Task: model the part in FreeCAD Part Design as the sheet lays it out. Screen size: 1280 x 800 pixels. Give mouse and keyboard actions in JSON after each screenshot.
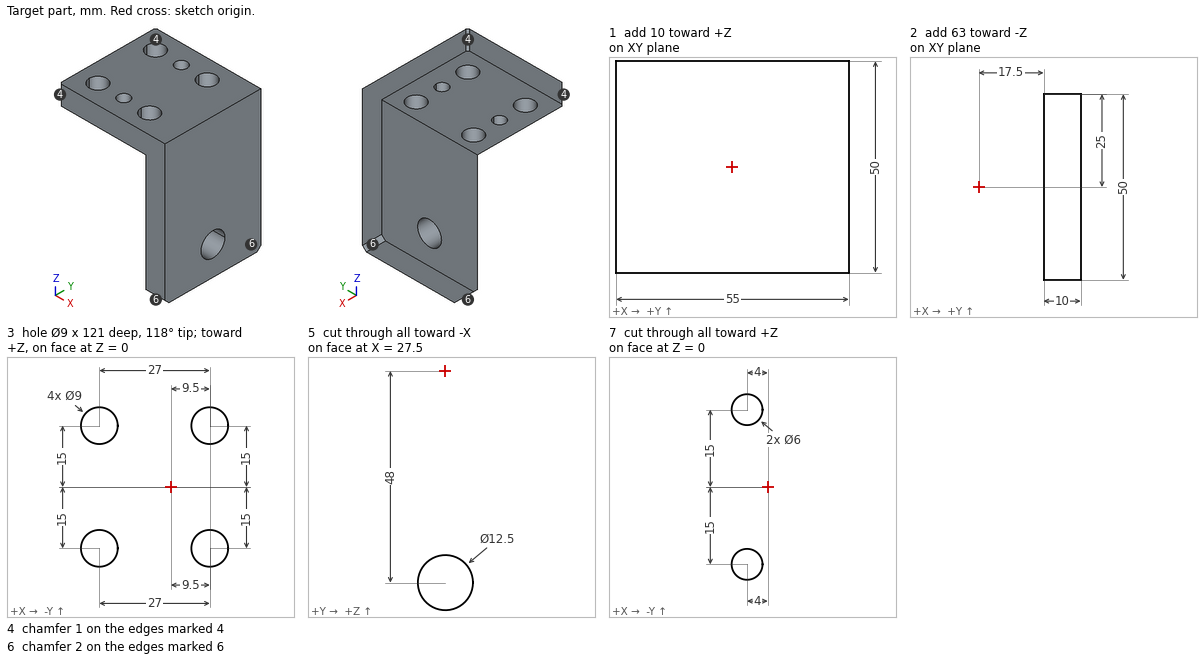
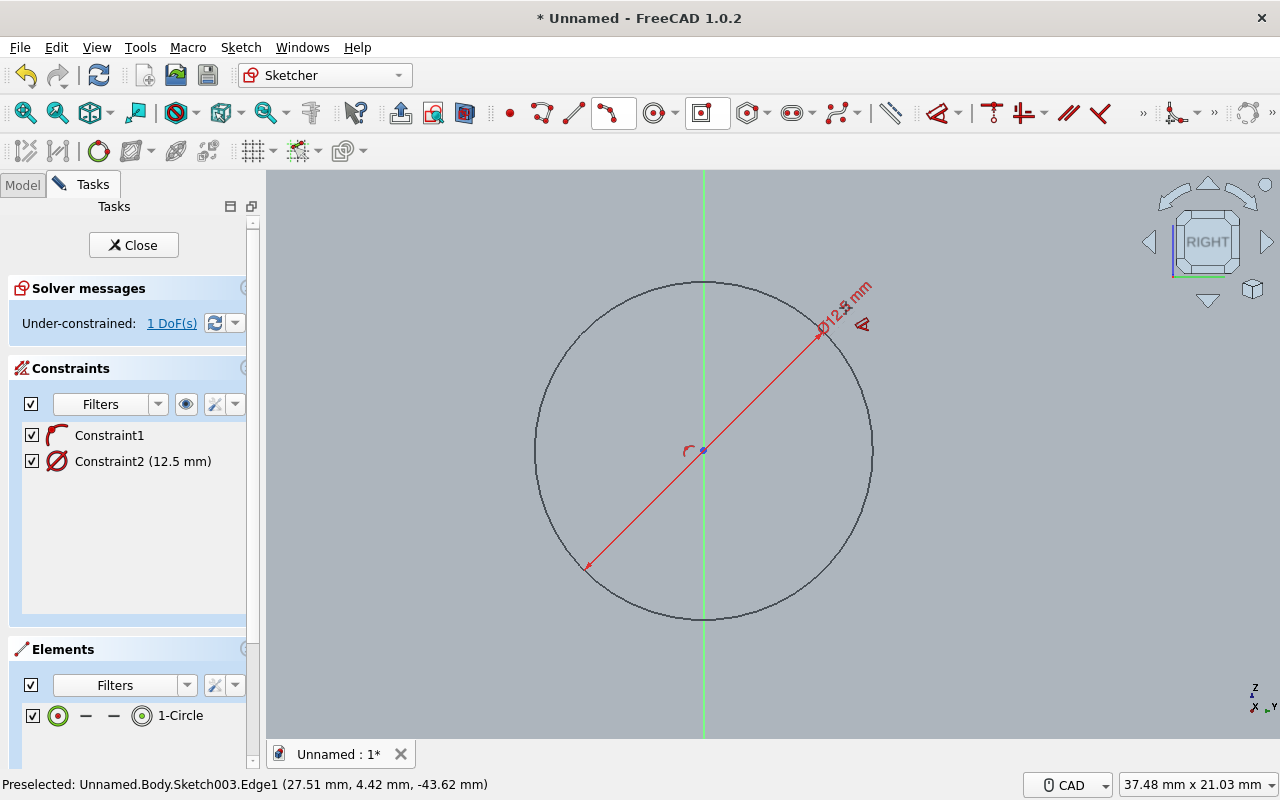
{"action": "left_click", "coordinate": [704, 451]}
{"action": "left_click", "coordinate": [738, 325]}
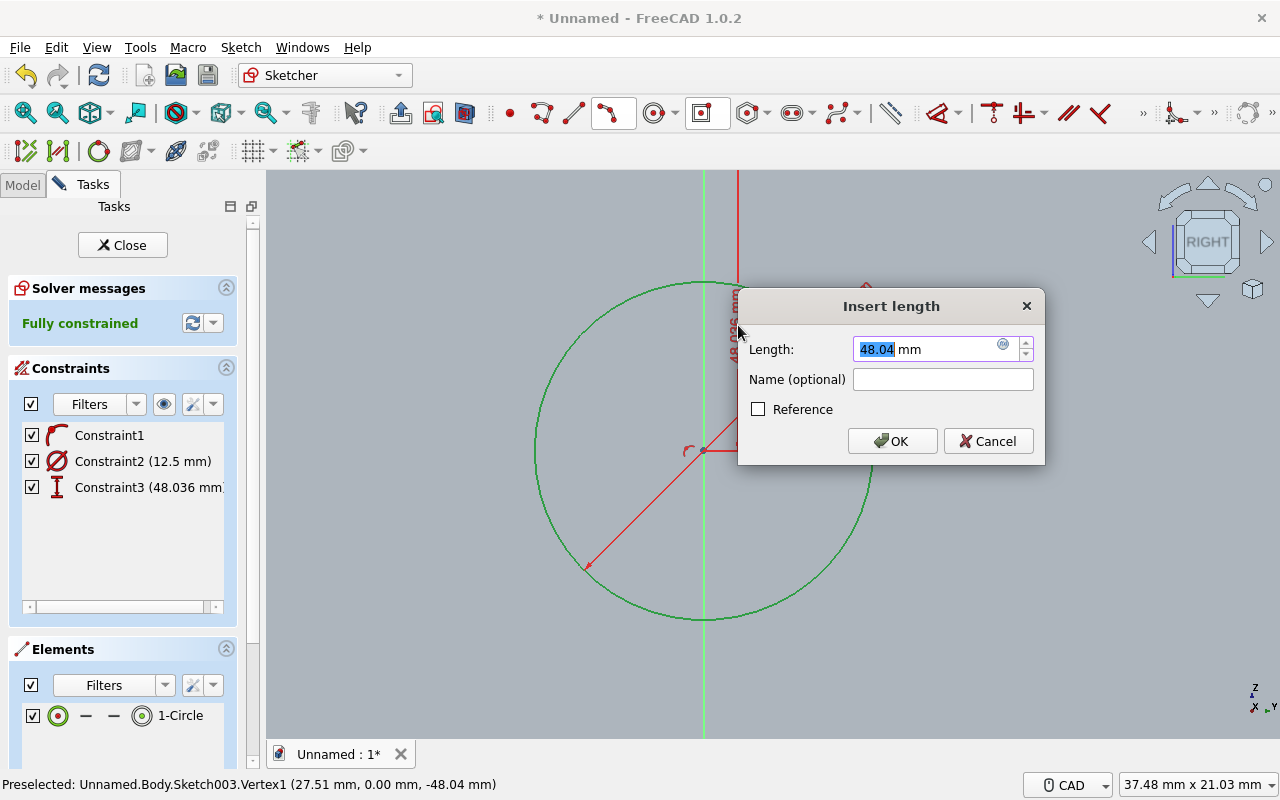
{"action": "type", "text": "48"}
{"action": "key", "text": "Return"}
{"action": "key", "text": "Escape"}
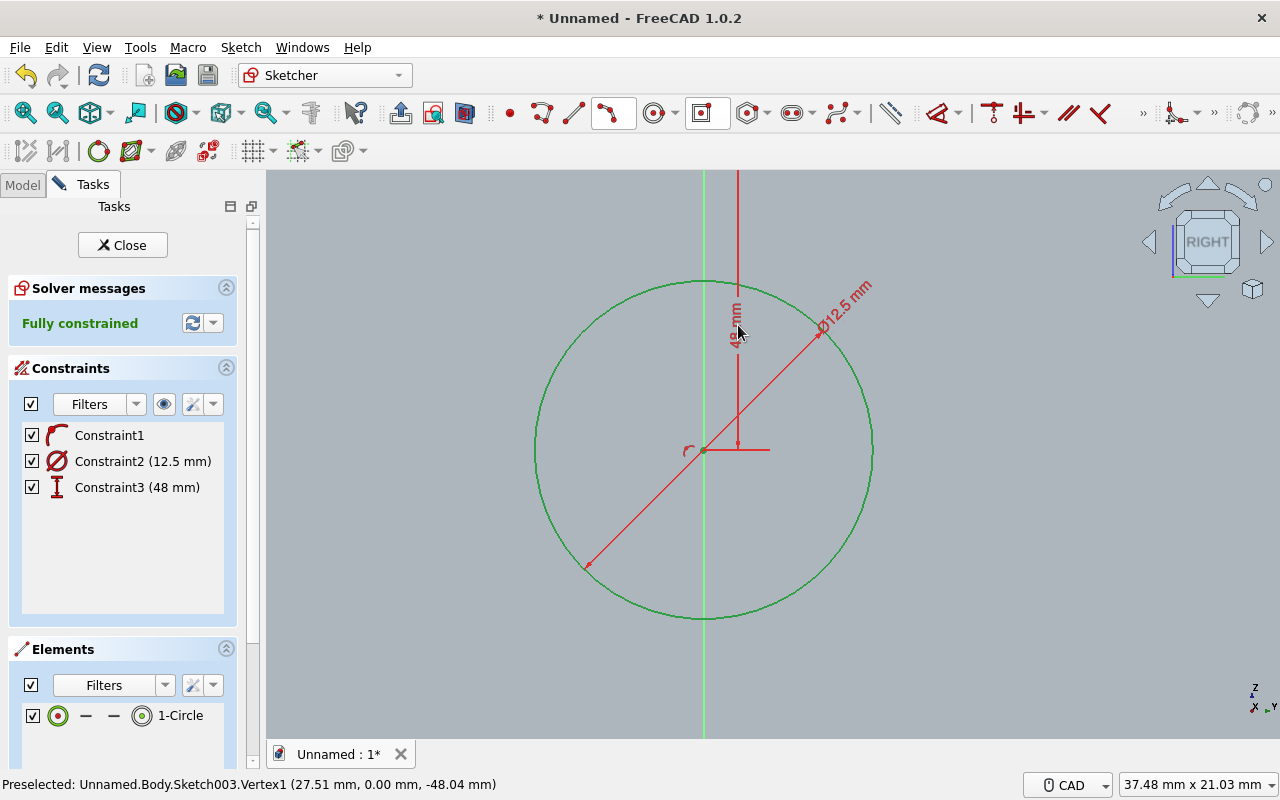
{"action": "left_click", "coordinate": [123, 245]}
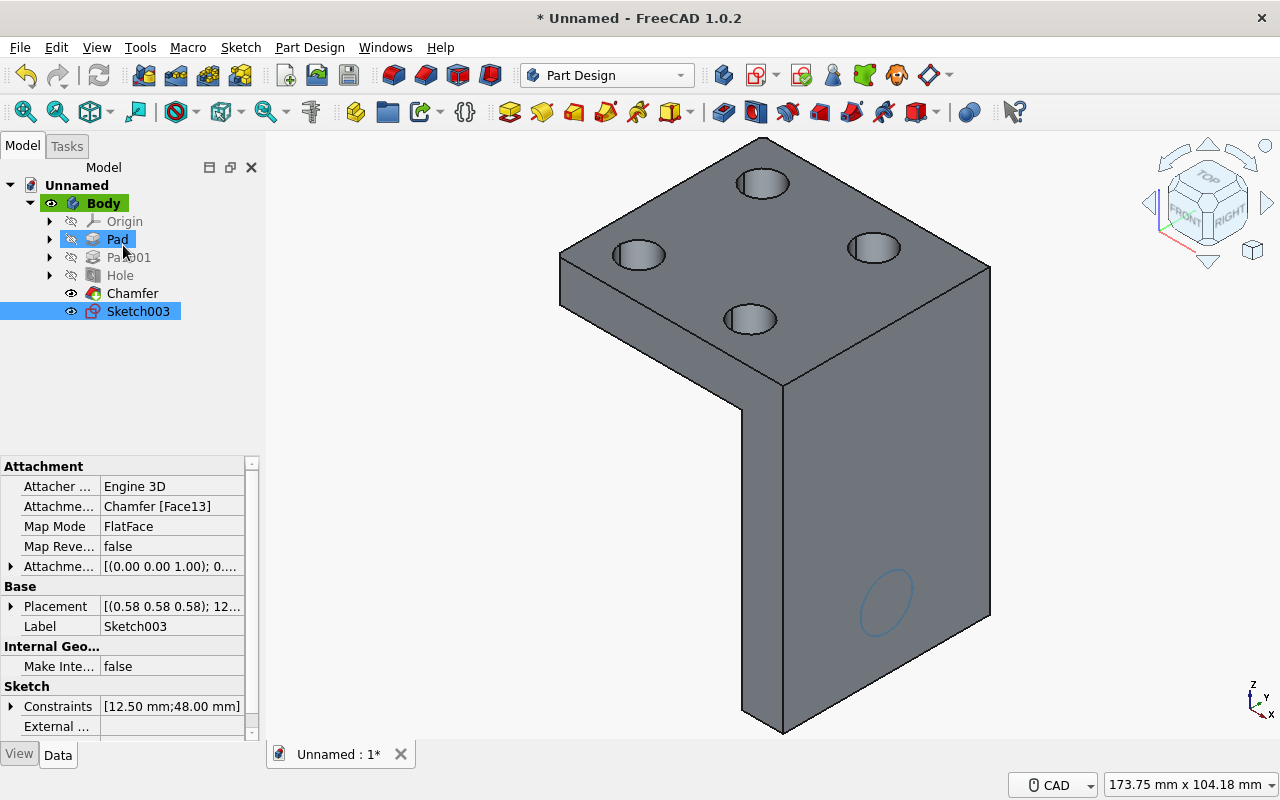
{"action": "left_click", "coordinate": [724, 112]}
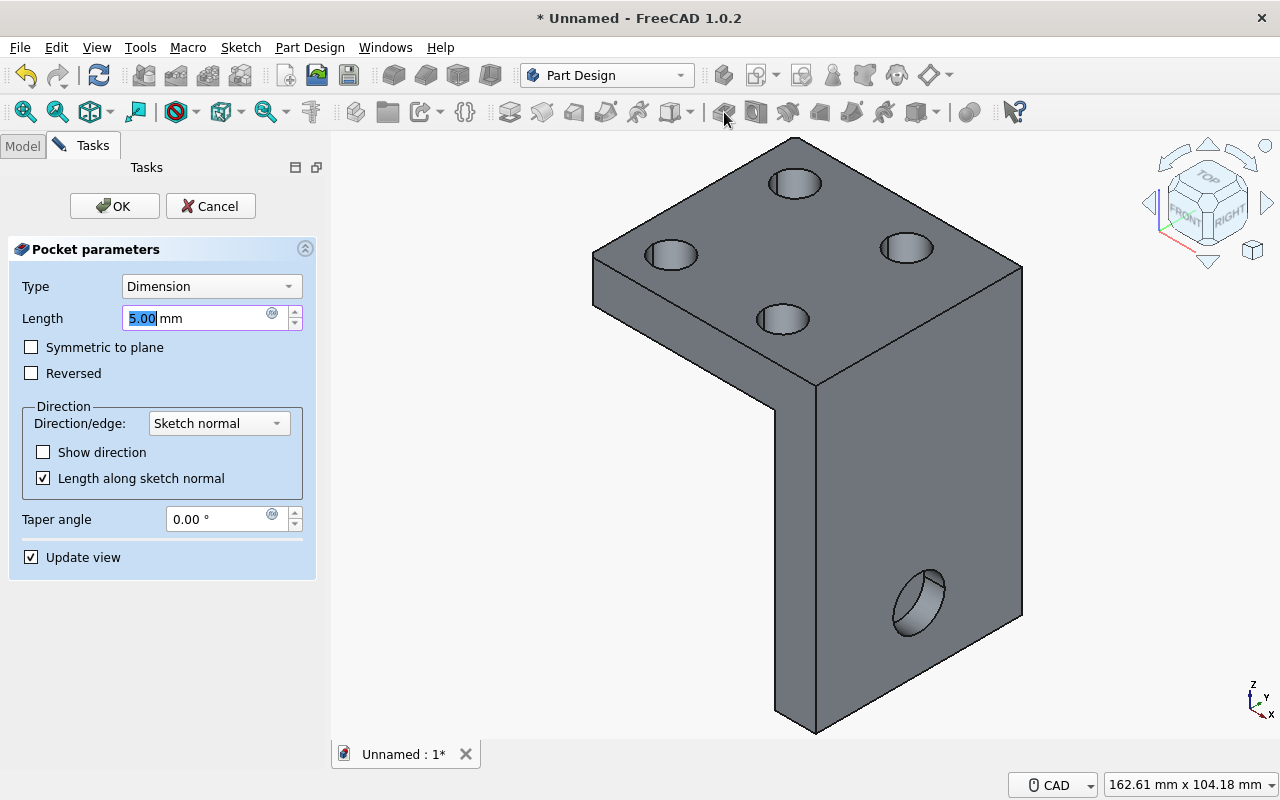
{"action": "left_click", "coordinate": [212, 286]}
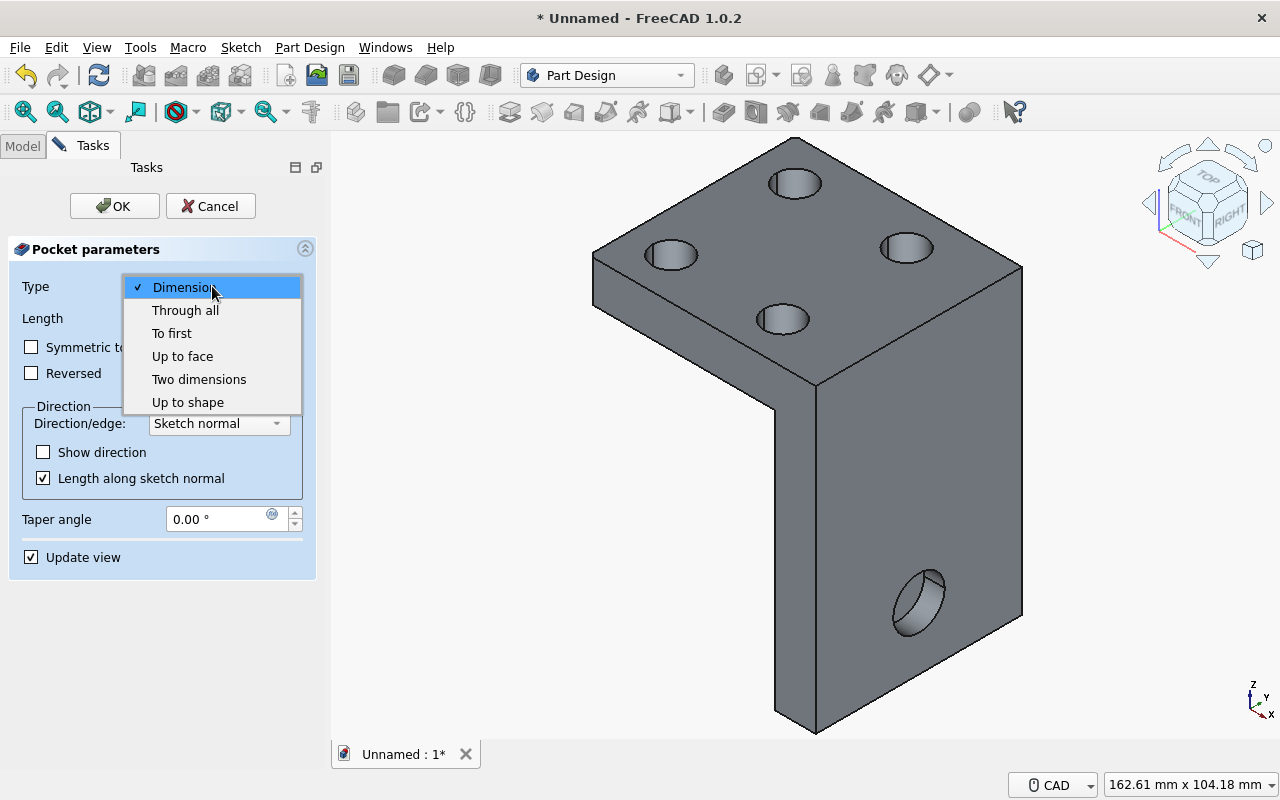
{"action": "left_click", "coordinate": [212, 310]}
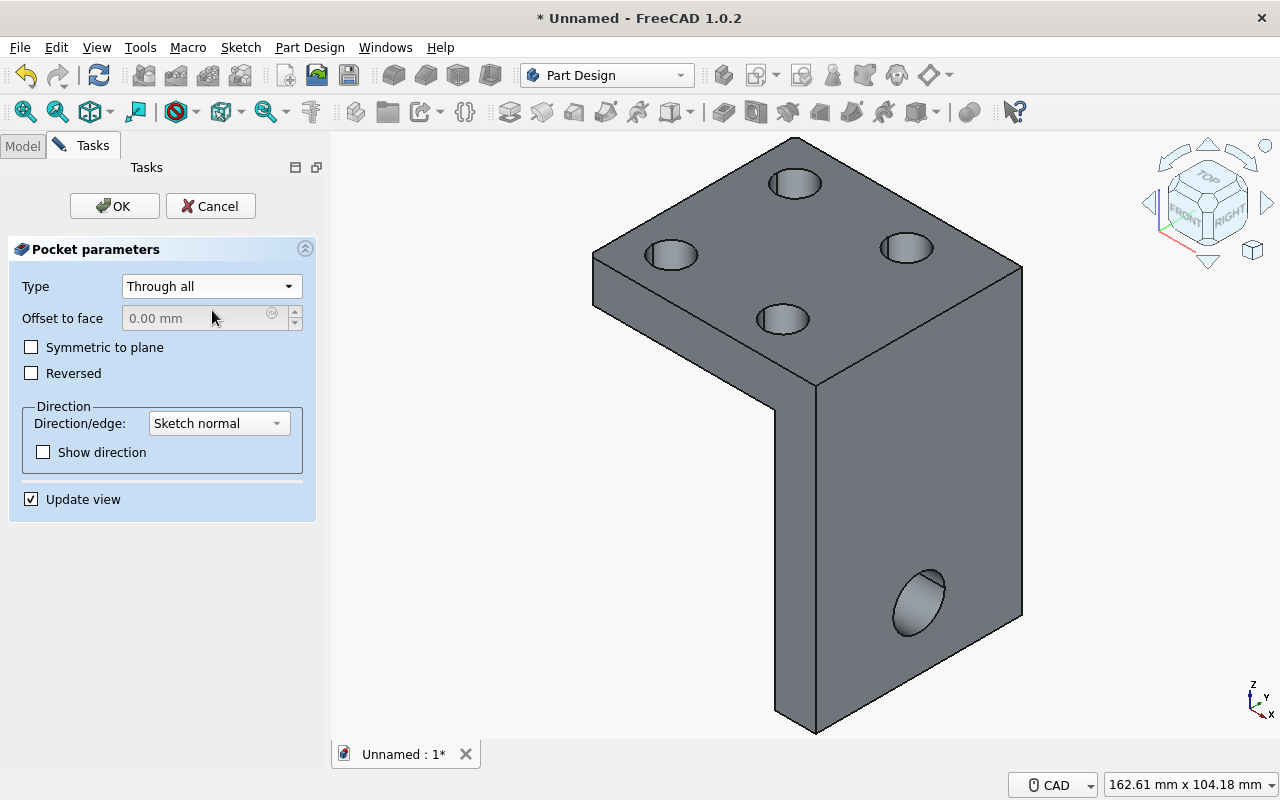
{"action": "left_click", "coordinate": [115, 206]}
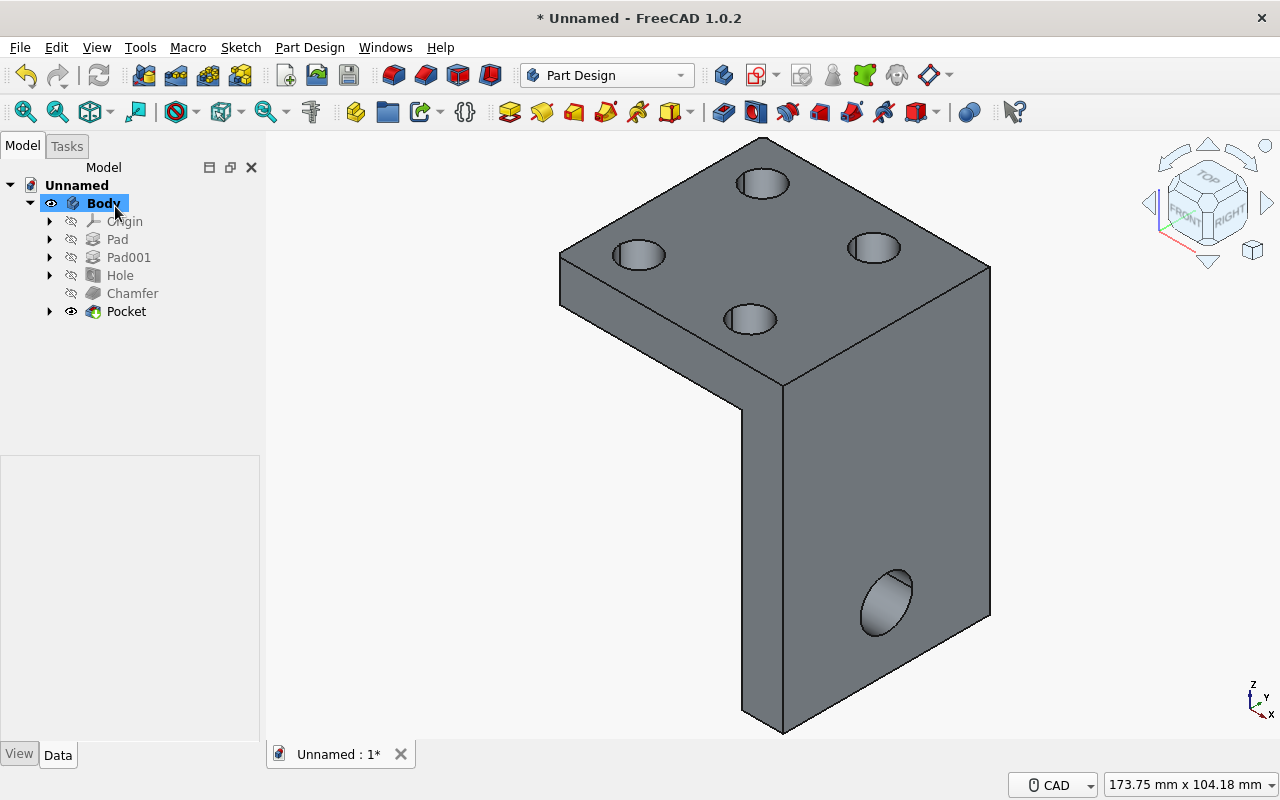
{"action": "key", "text": "2"}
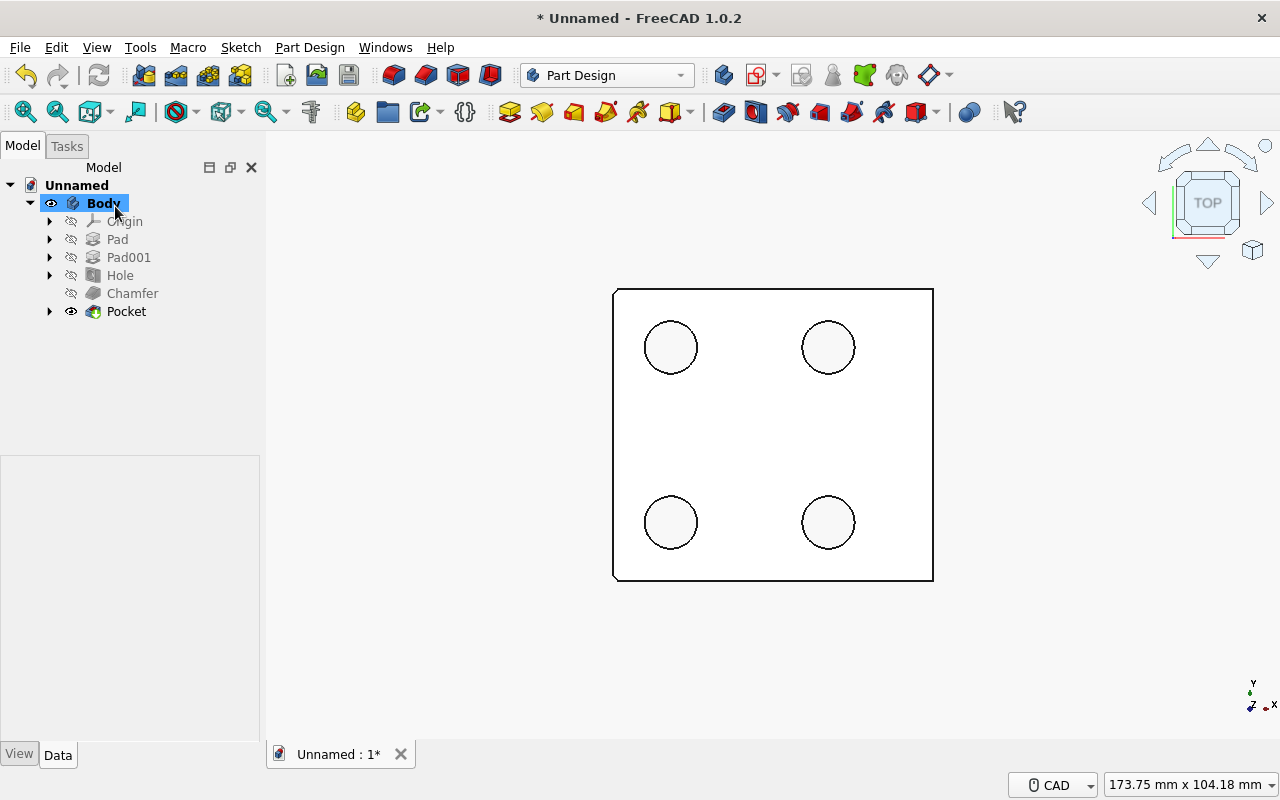
{"action": "key", "text": "0"}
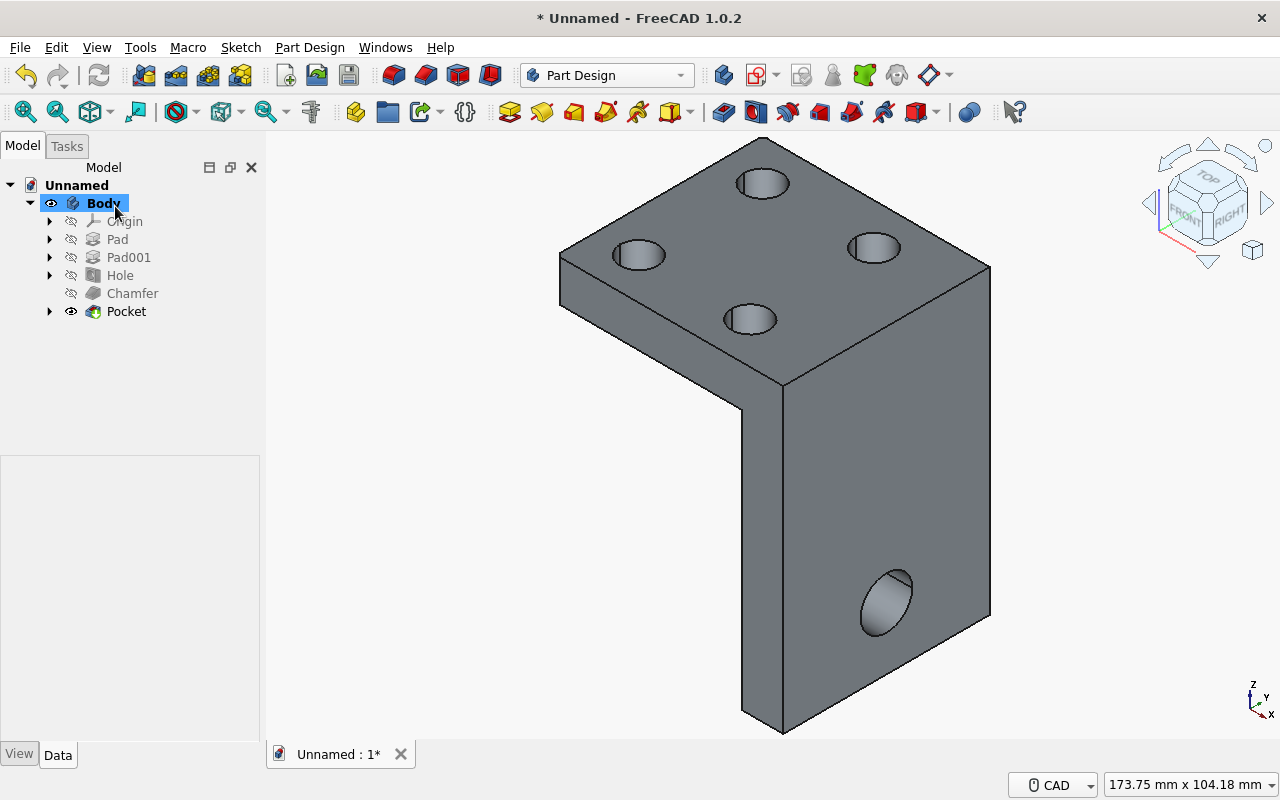
{"action": "key", "text": "1"}